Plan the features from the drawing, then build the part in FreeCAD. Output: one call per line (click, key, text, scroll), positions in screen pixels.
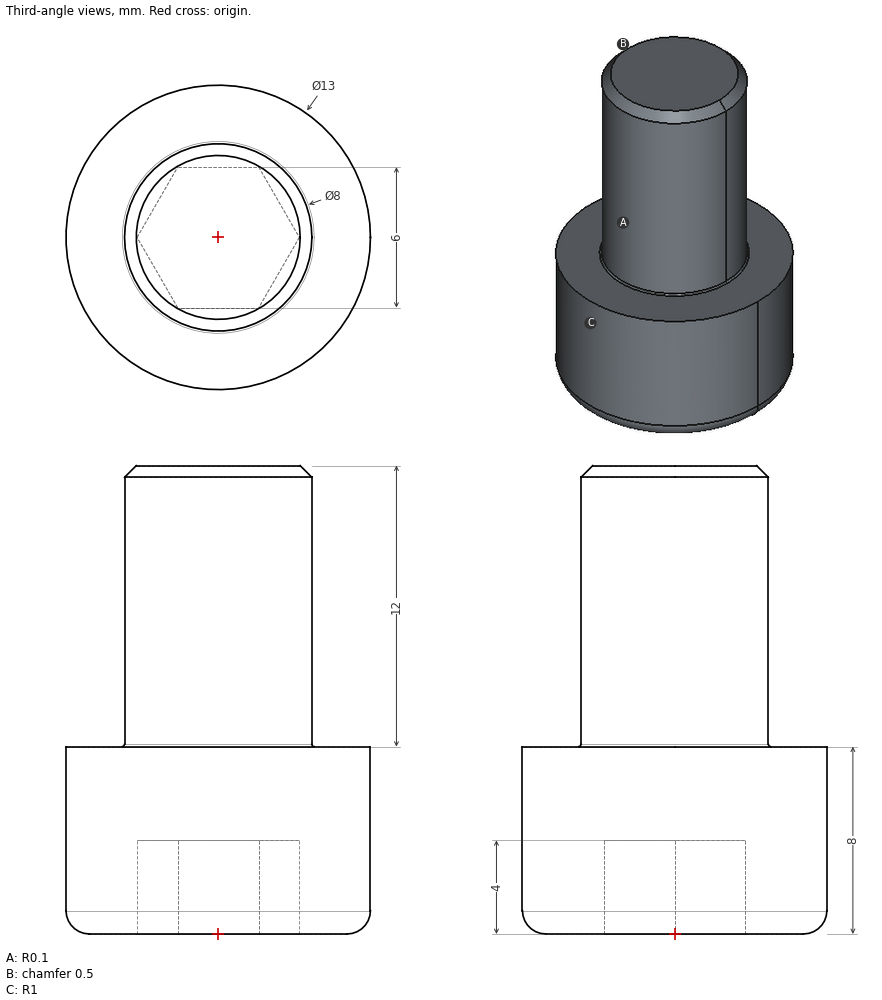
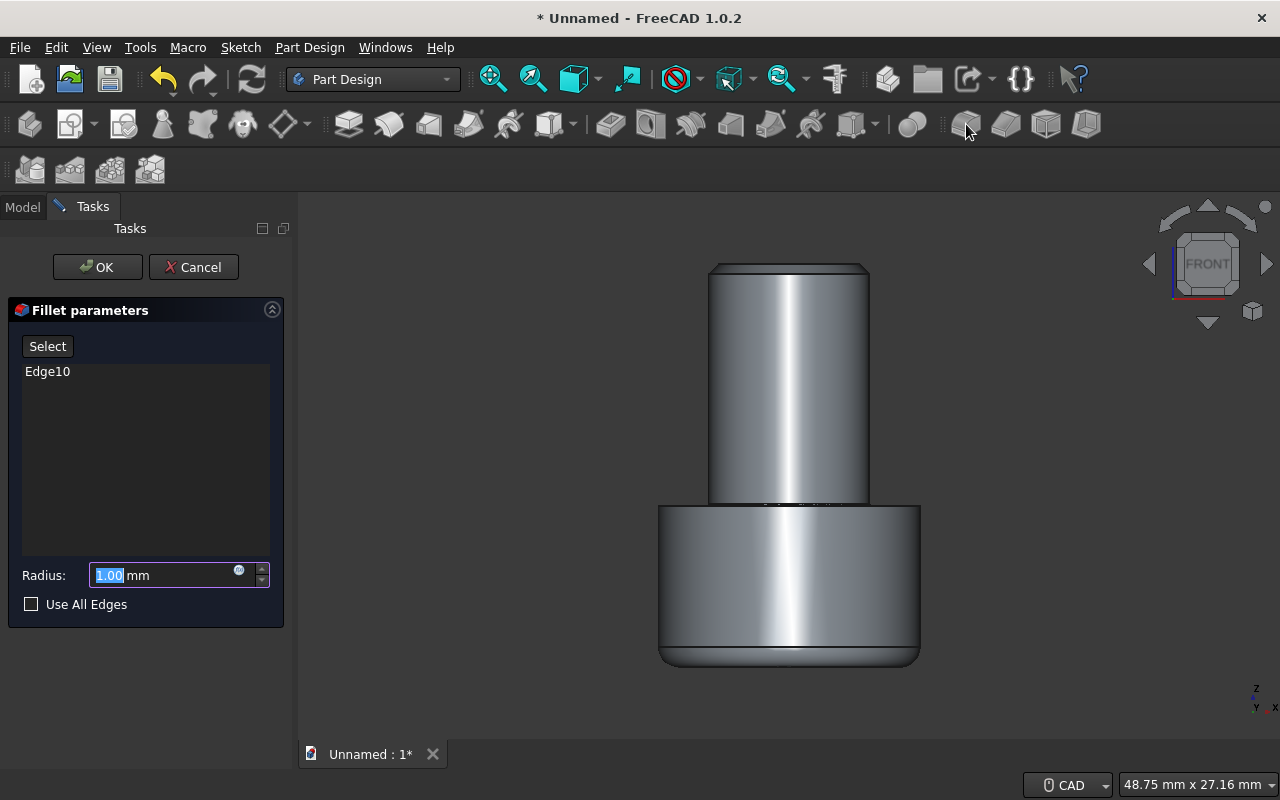
text(1)
key(Tab)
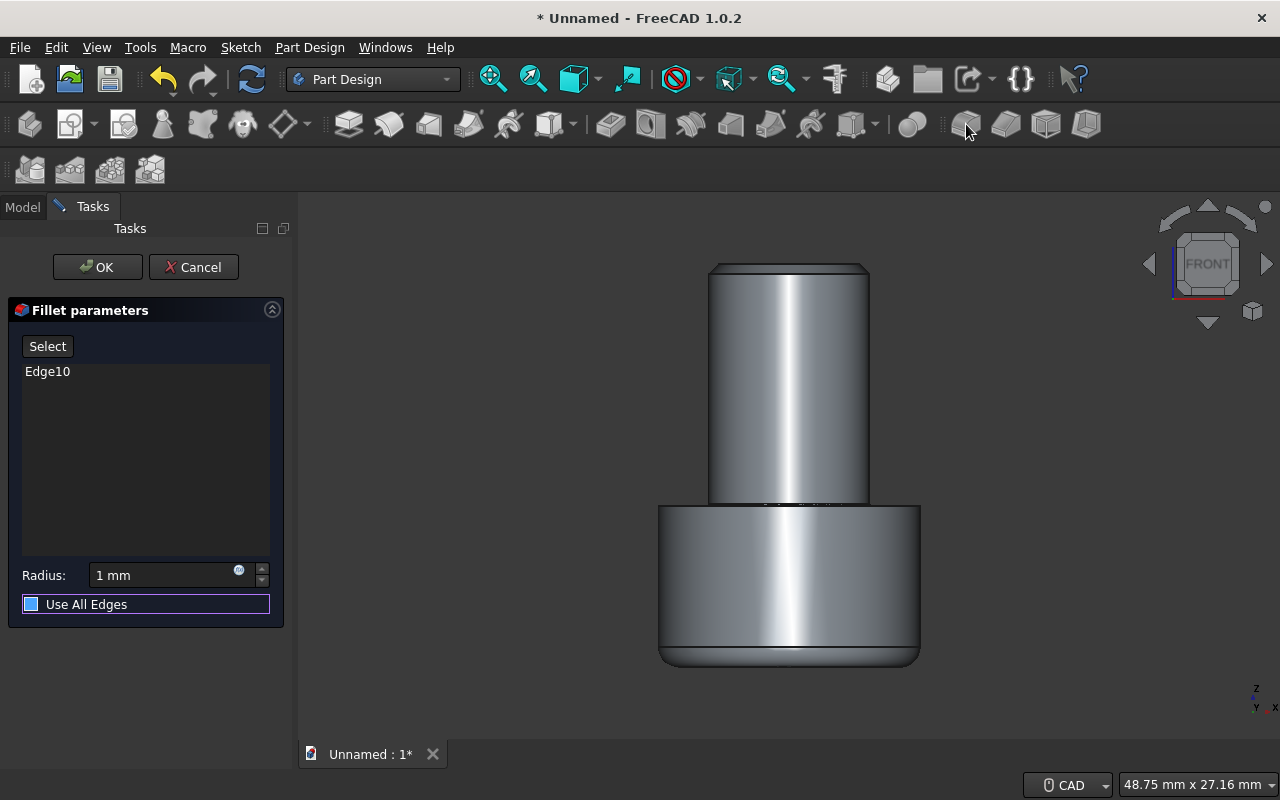
click(98, 267)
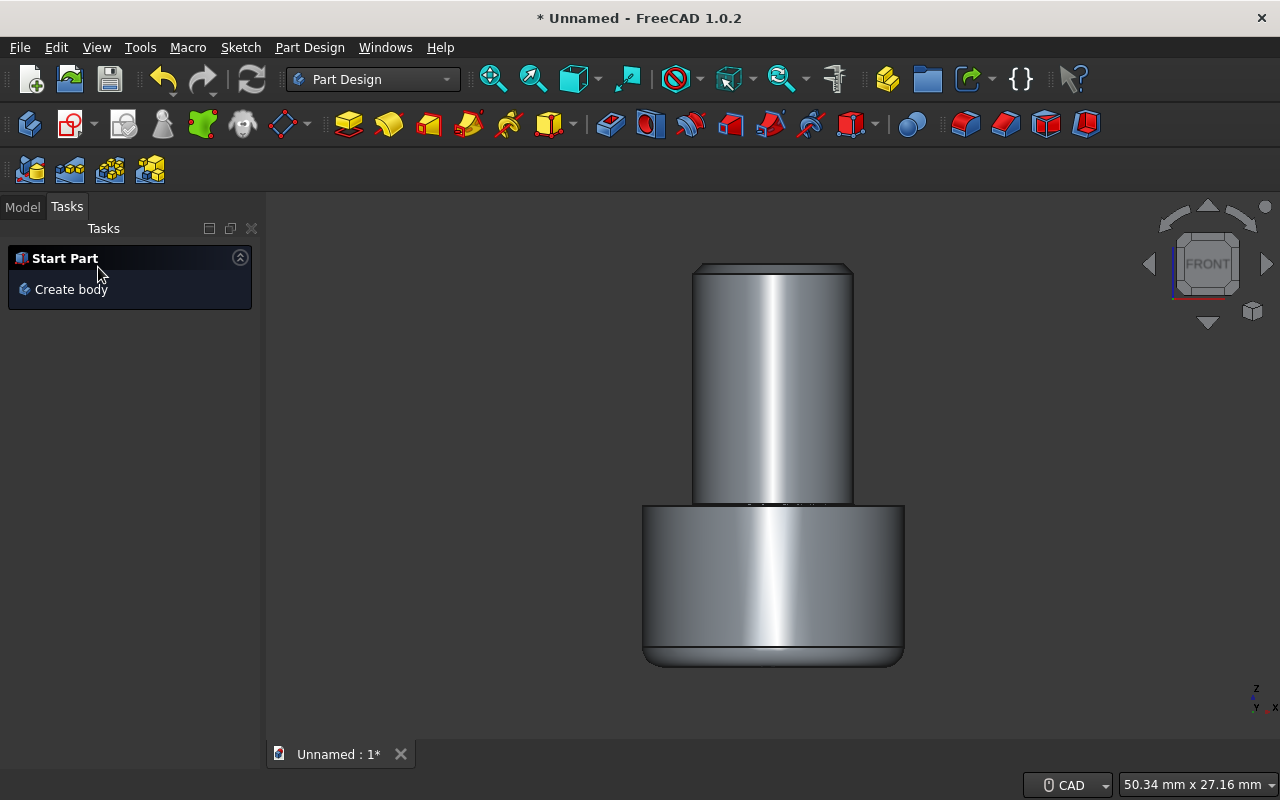
key(0)